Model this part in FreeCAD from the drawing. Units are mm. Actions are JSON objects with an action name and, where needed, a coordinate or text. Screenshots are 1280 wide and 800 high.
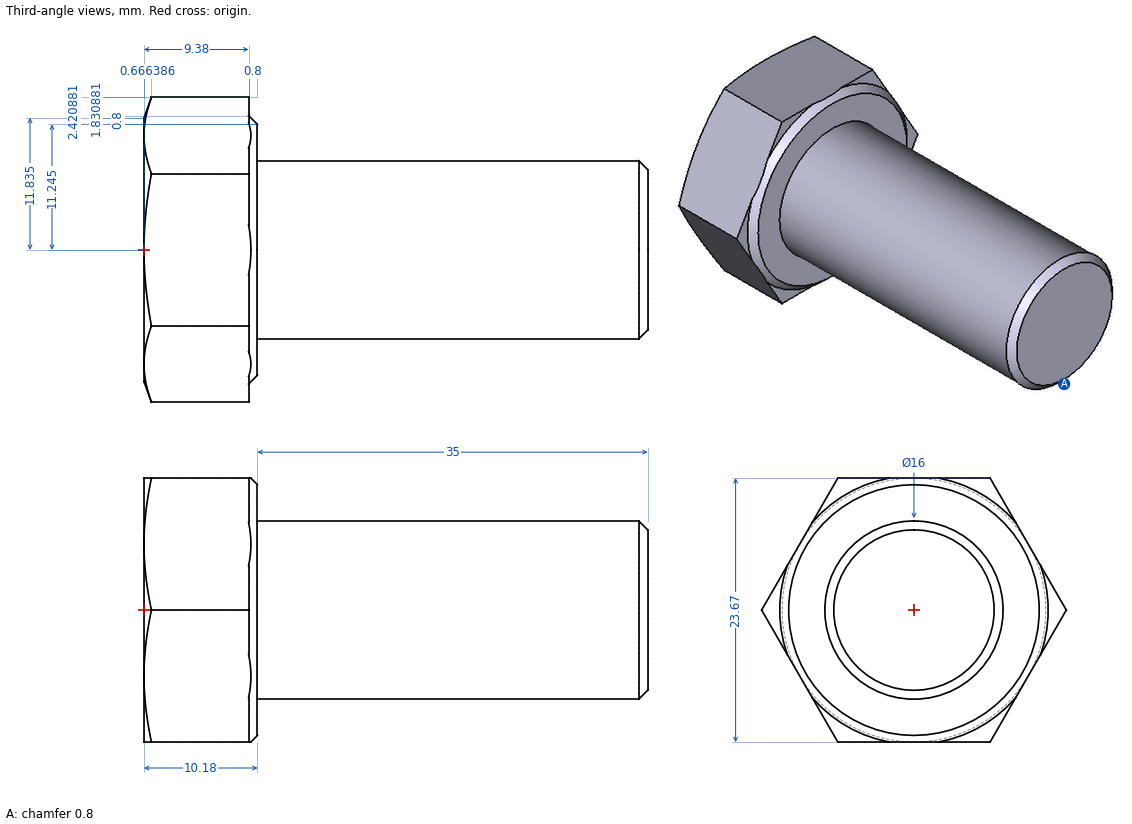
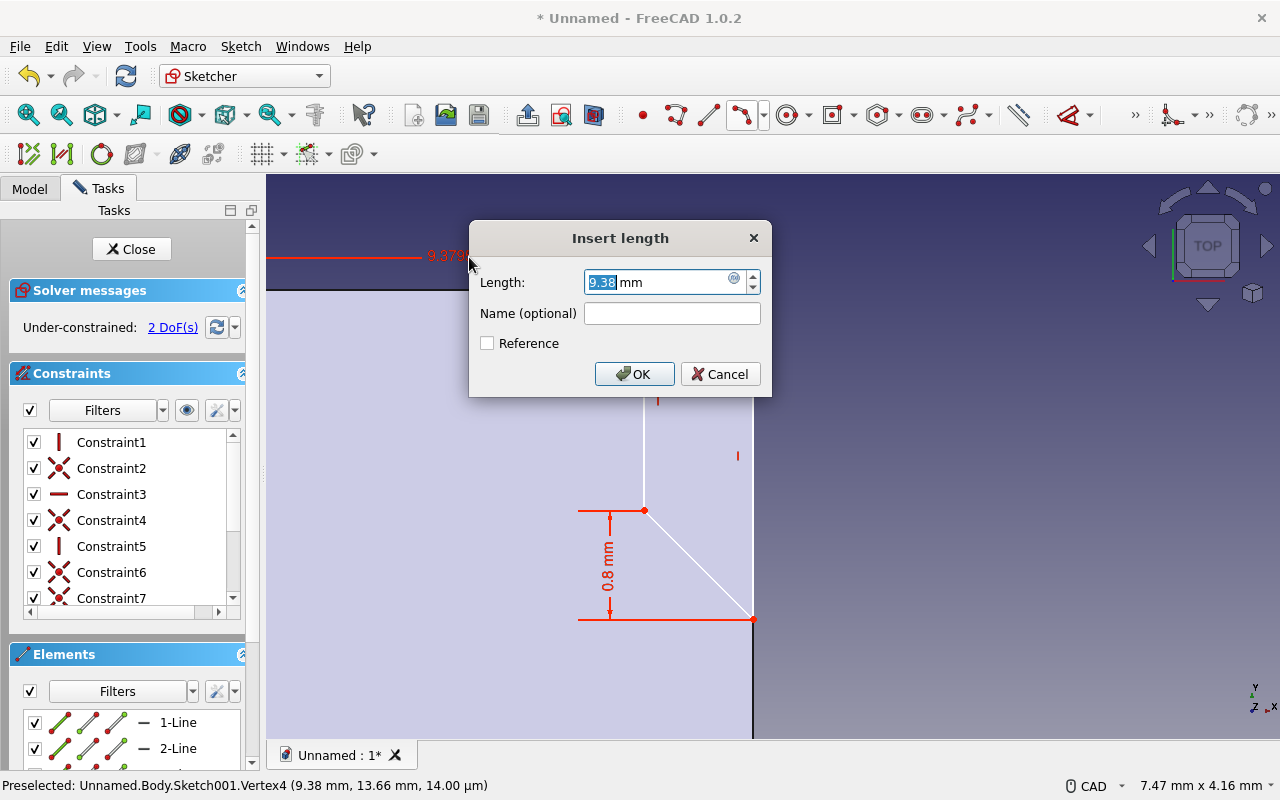
{"action": "type", "text": "9.38"}
{"action": "key", "text": "Return"}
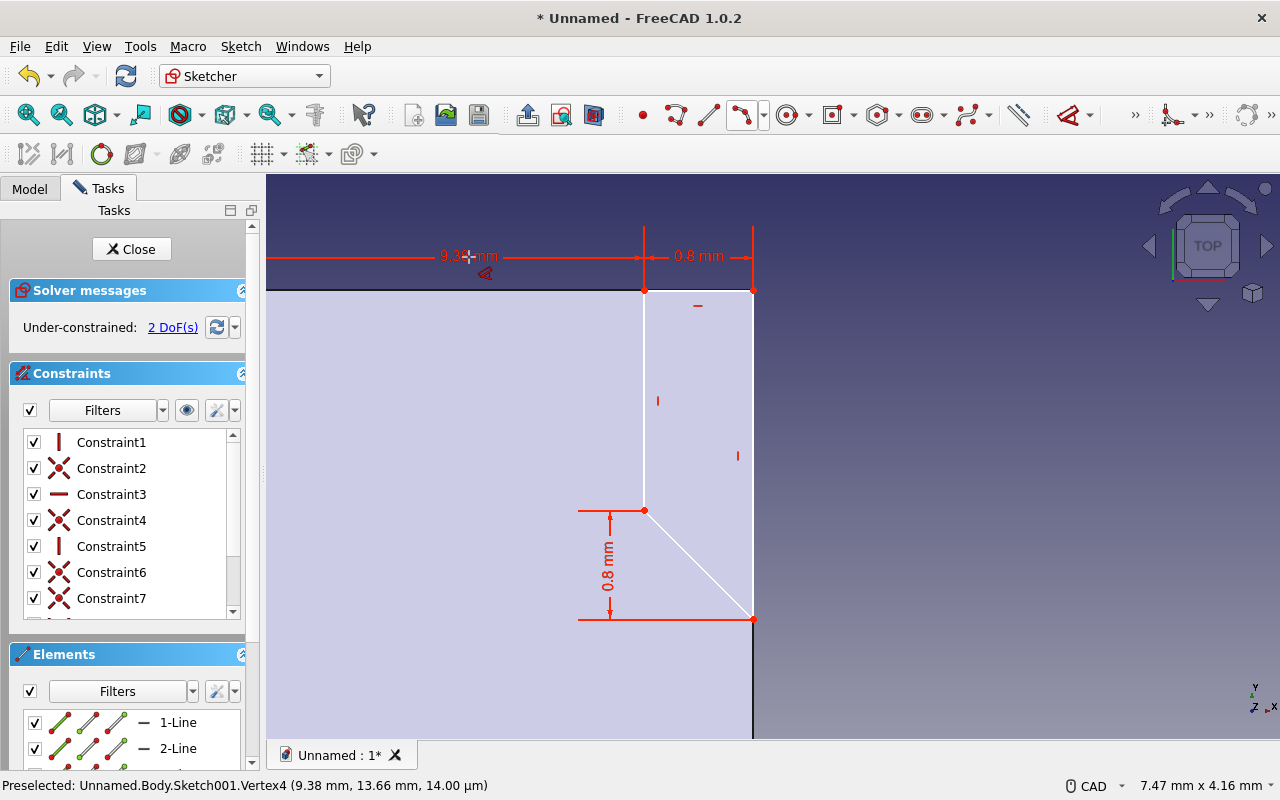
{"action": "left_click", "coordinate": [753, 620]}
{"action": "left_click", "coordinate": [787, 665]}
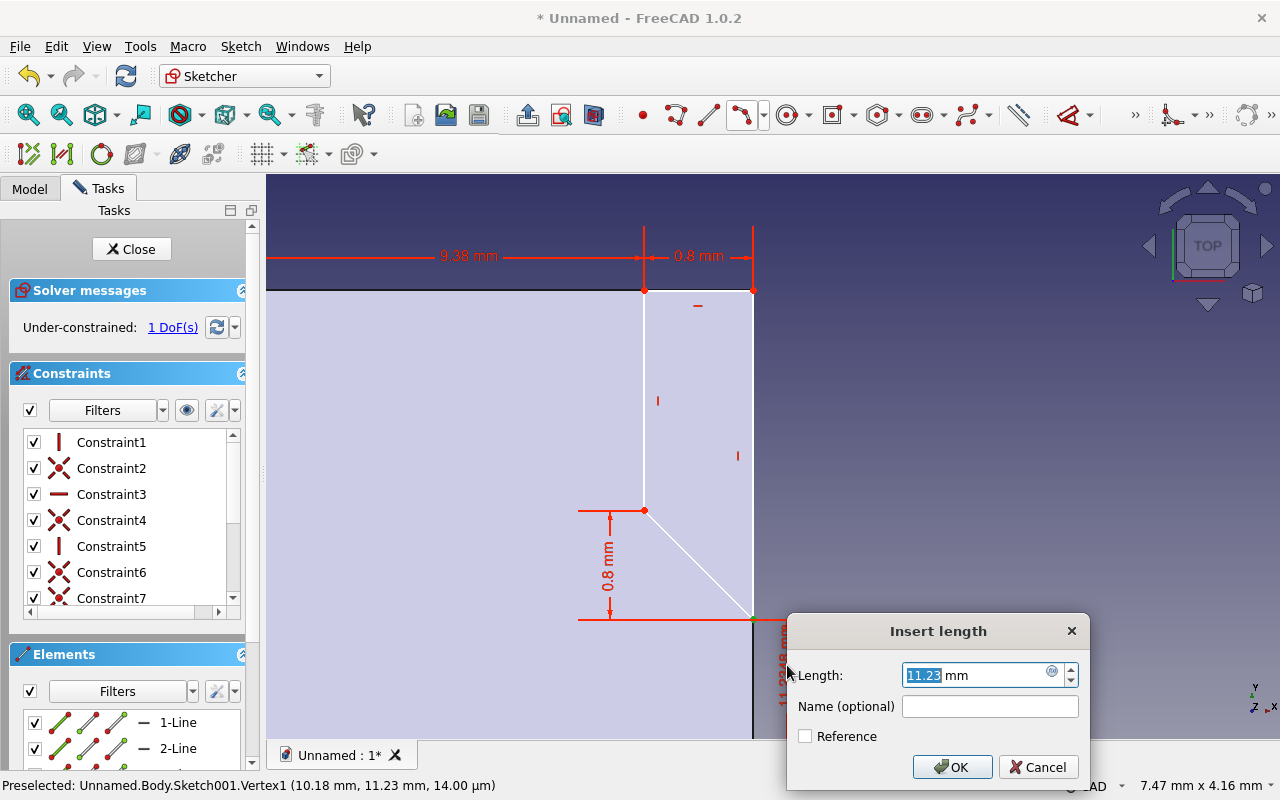
{"action": "type", "text": "11.245"}
{"action": "key", "text": "Return"}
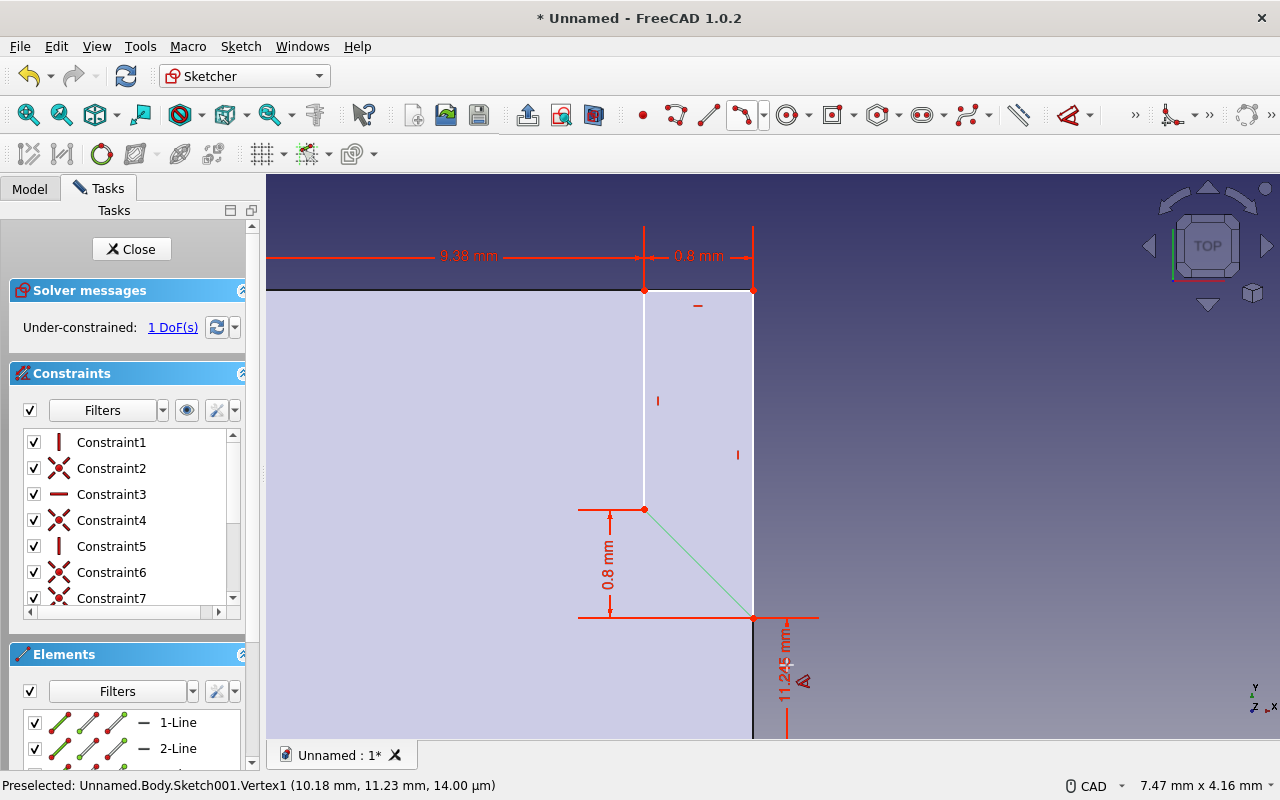
{"action": "left_click", "coordinate": [753, 520]}
{"action": "left_click", "coordinate": [787, 455]}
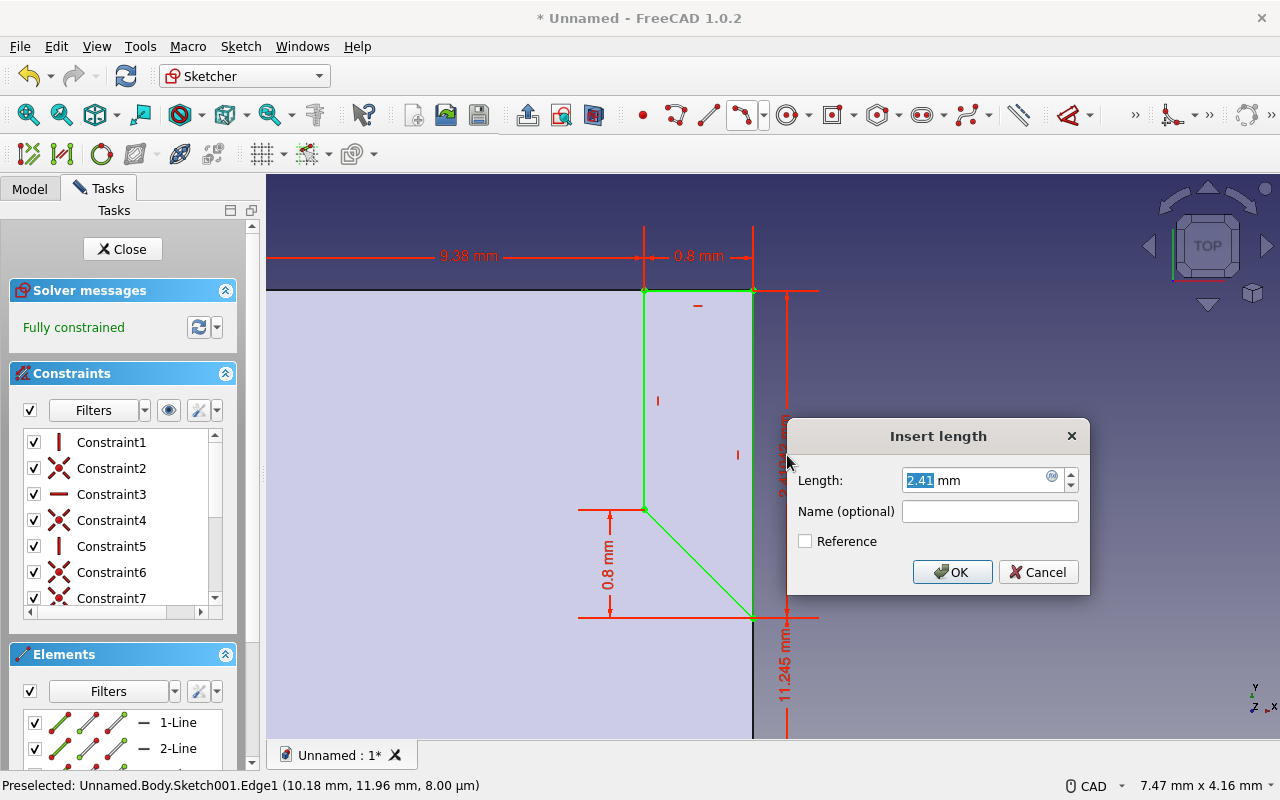
{"action": "type", "text": "2.420881"}
{"action": "key", "text": "Return"}
{"action": "key", "text": "Escape"}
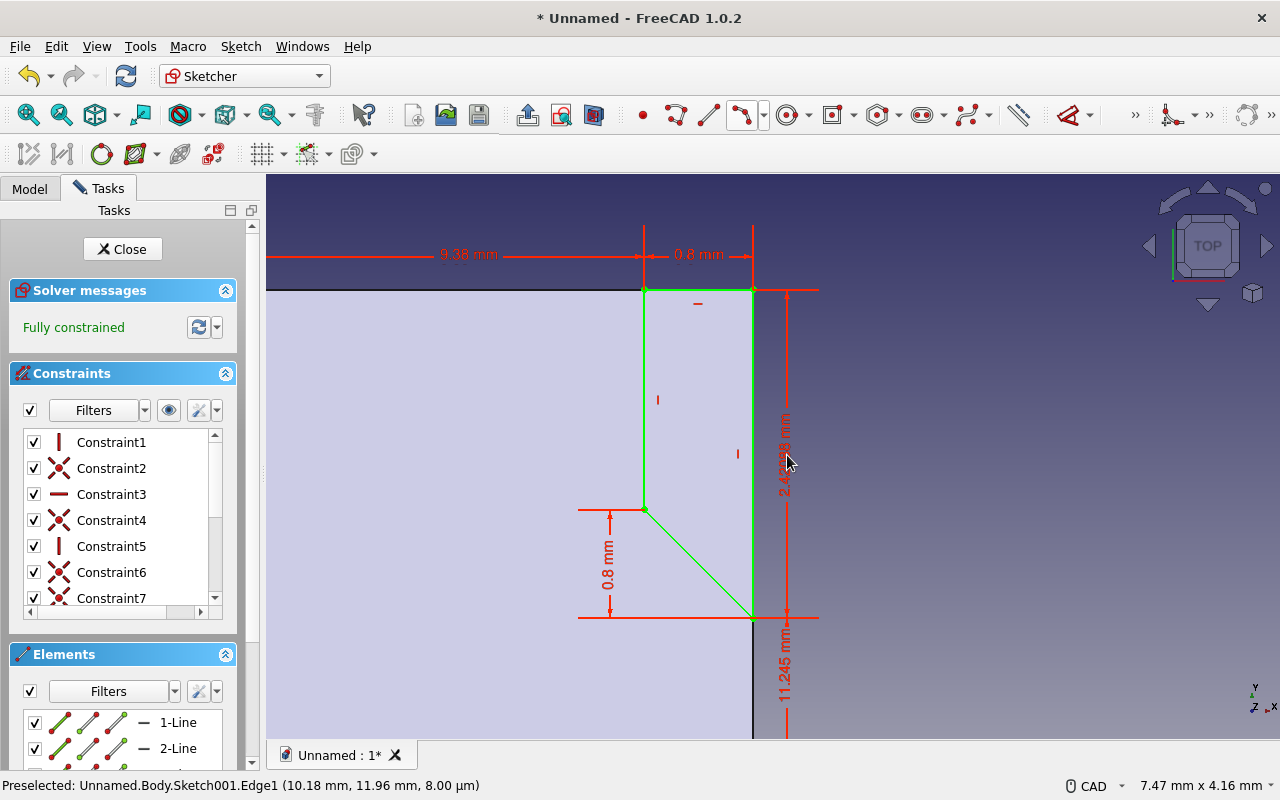
{"action": "left_click", "coordinate": [123, 249]}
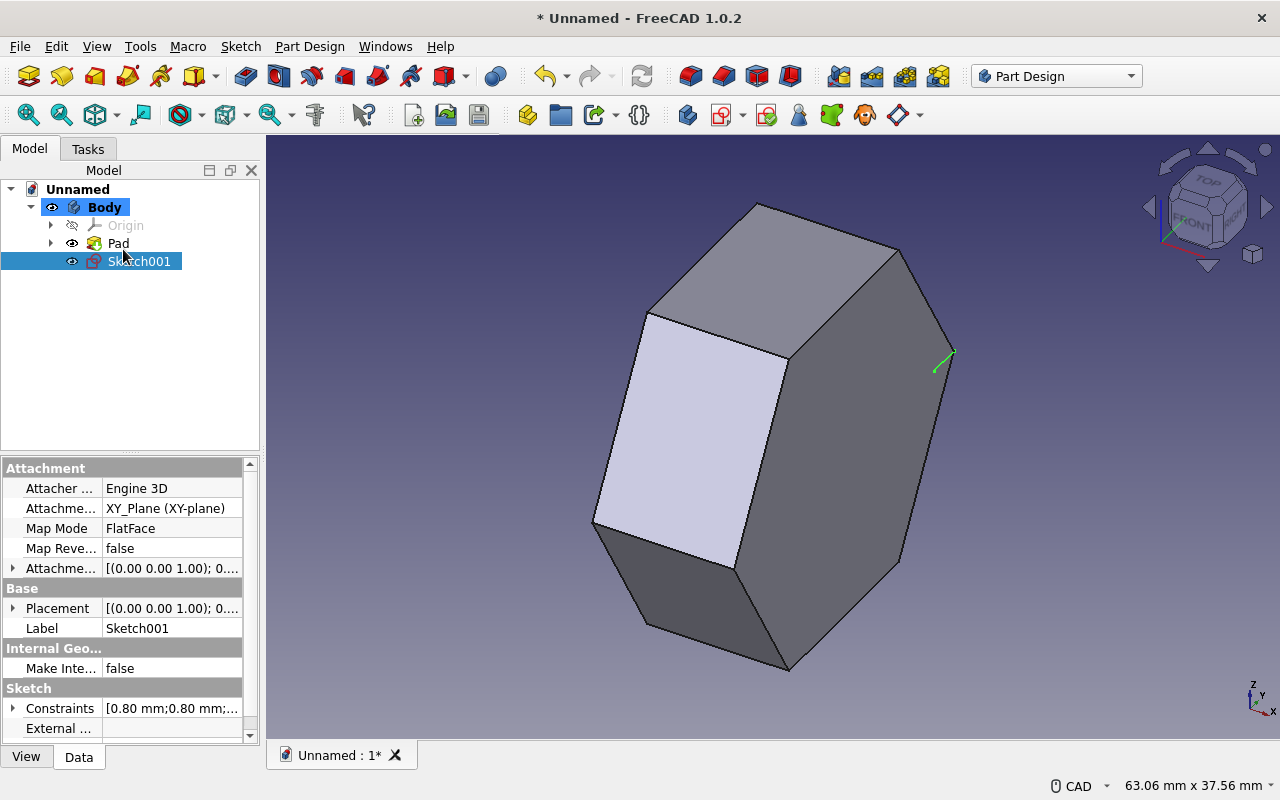
{"action": "left_click", "coordinate": [312, 76]}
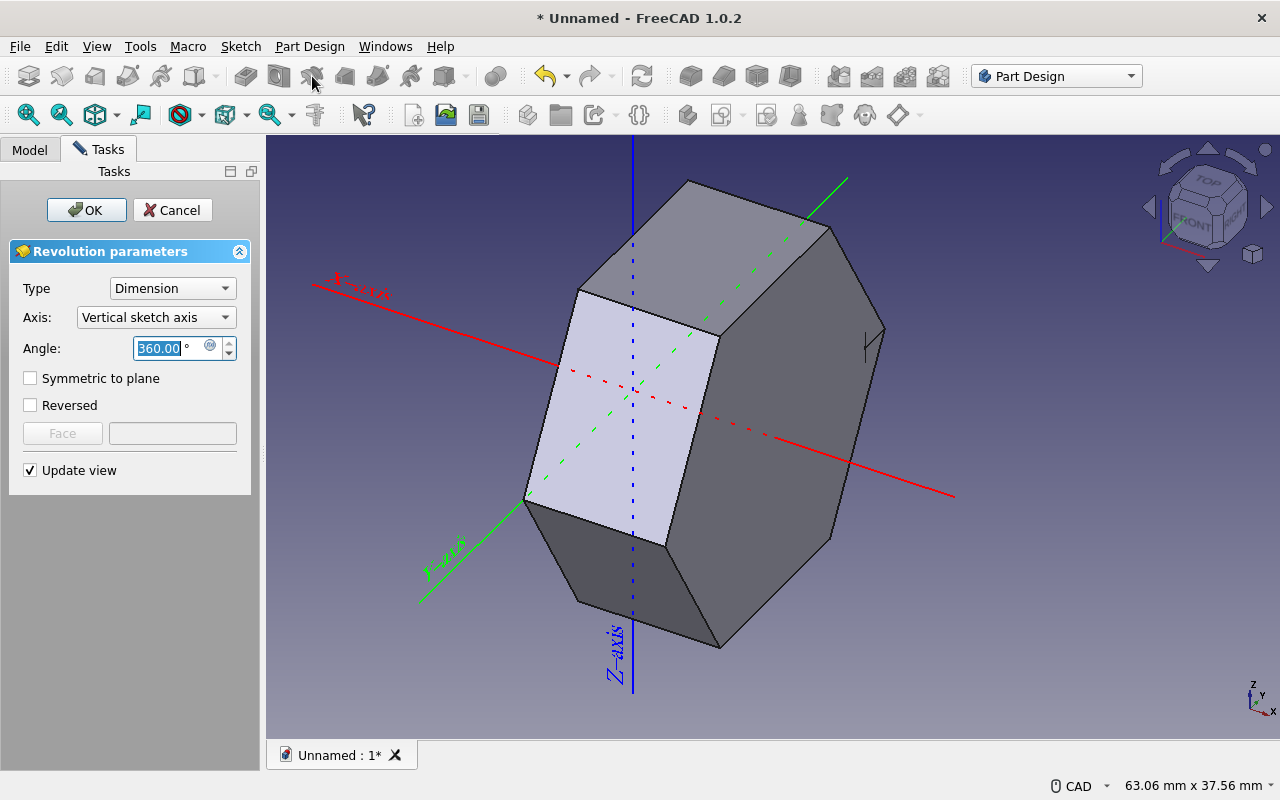
{"action": "left_click", "coordinate": [157, 318]}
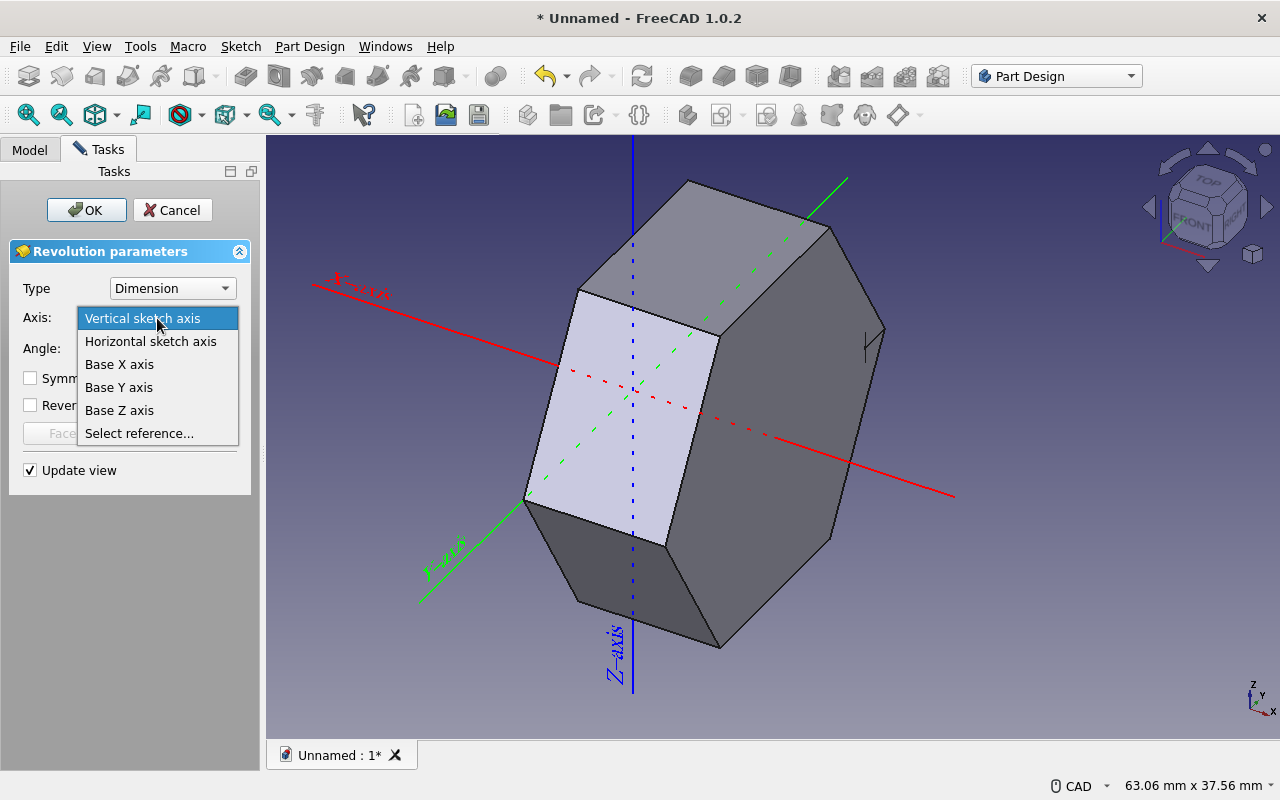
{"action": "left_click", "coordinate": [156, 342]}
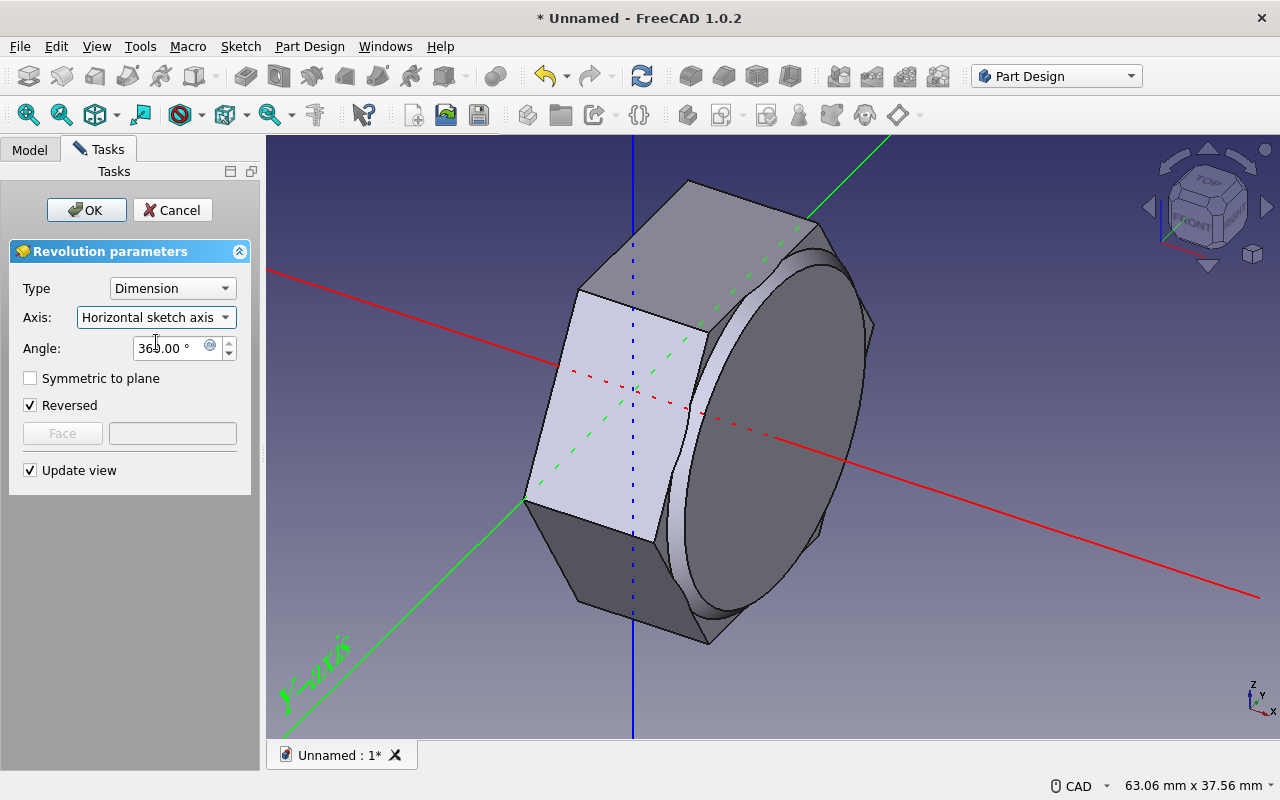
{"action": "left_click", "coordinate": [87, 210]}